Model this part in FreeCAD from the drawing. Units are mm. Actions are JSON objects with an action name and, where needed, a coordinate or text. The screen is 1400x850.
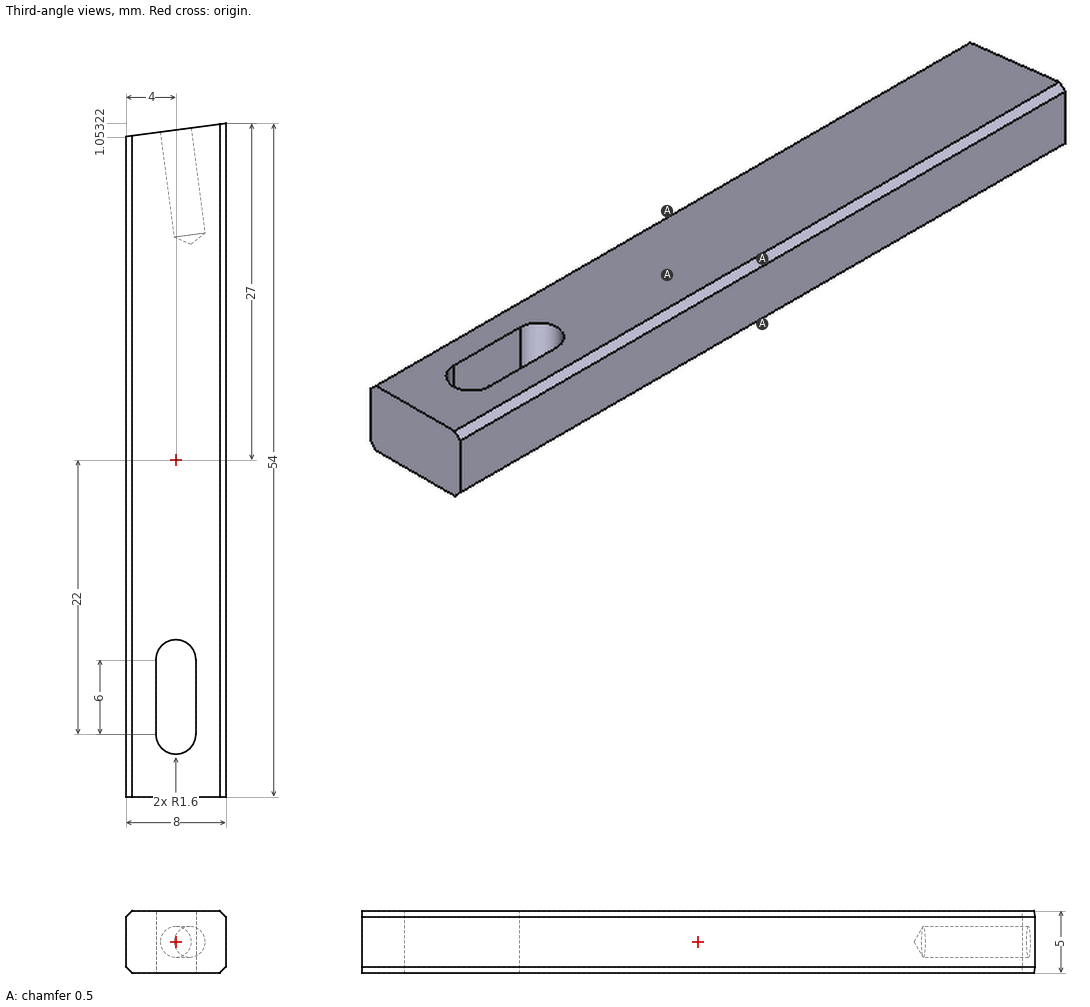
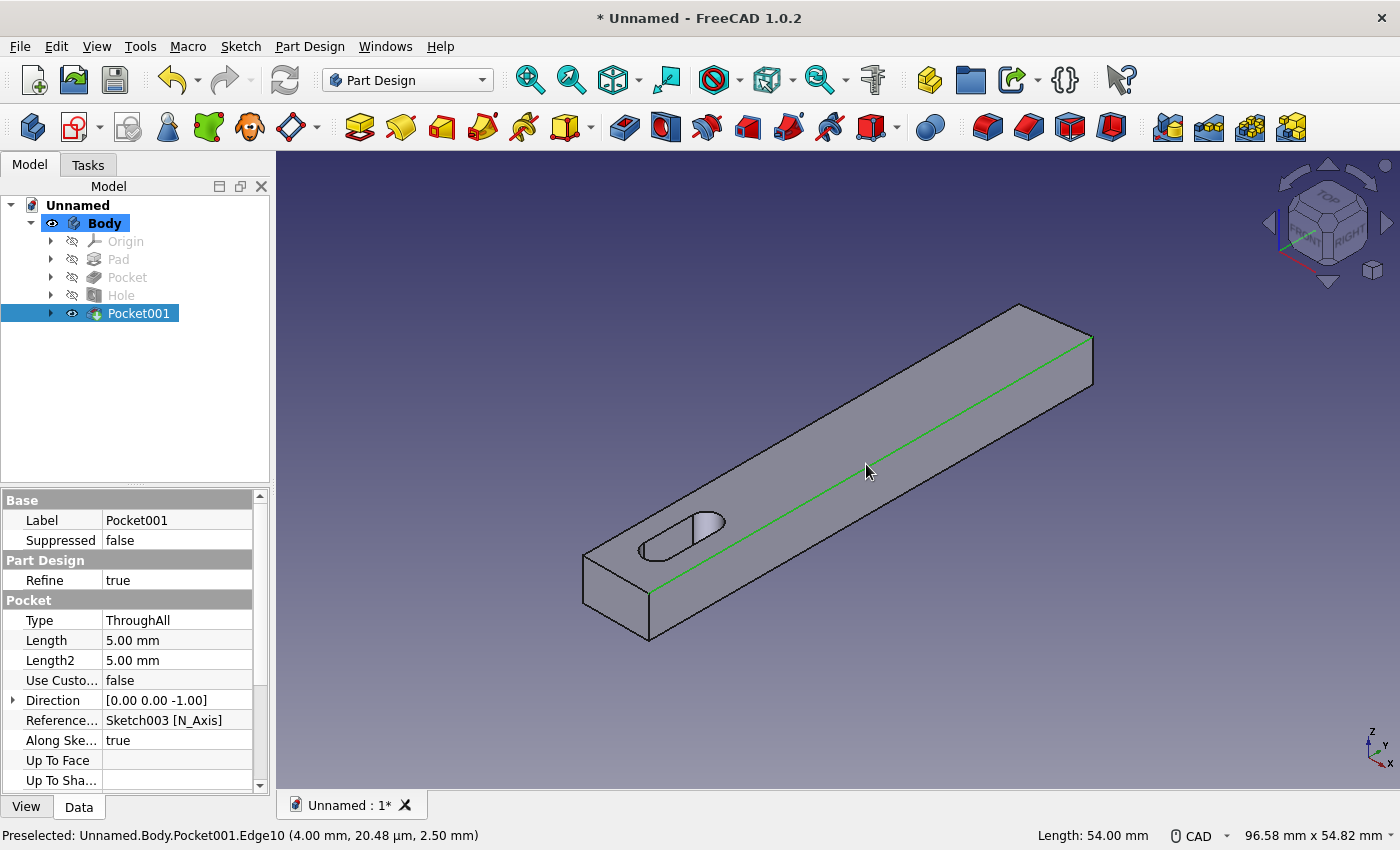
{"action": "key", "text": "2"}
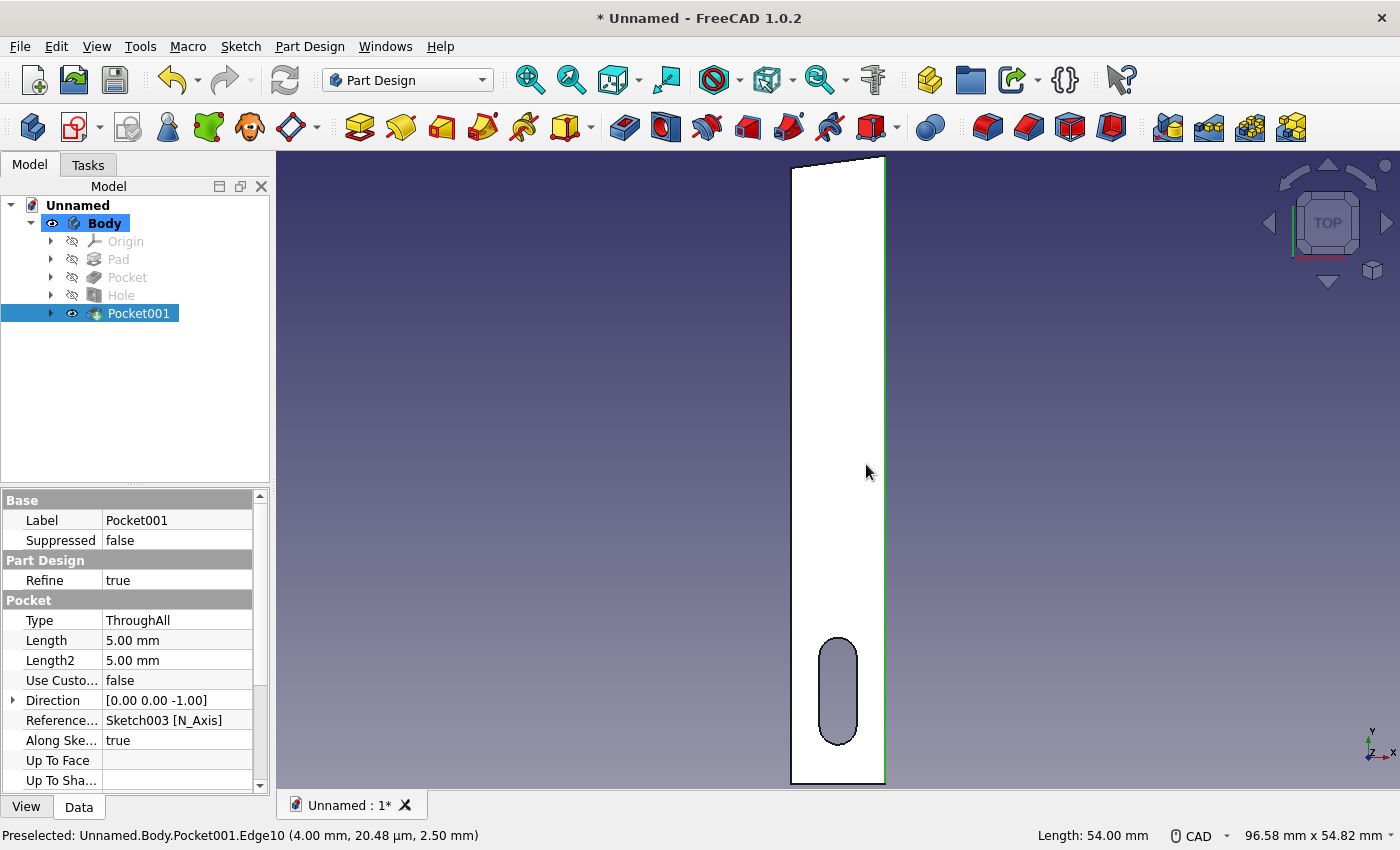
{"action": "left_click", "coordinate": [791, 475], "text": "ctrl"}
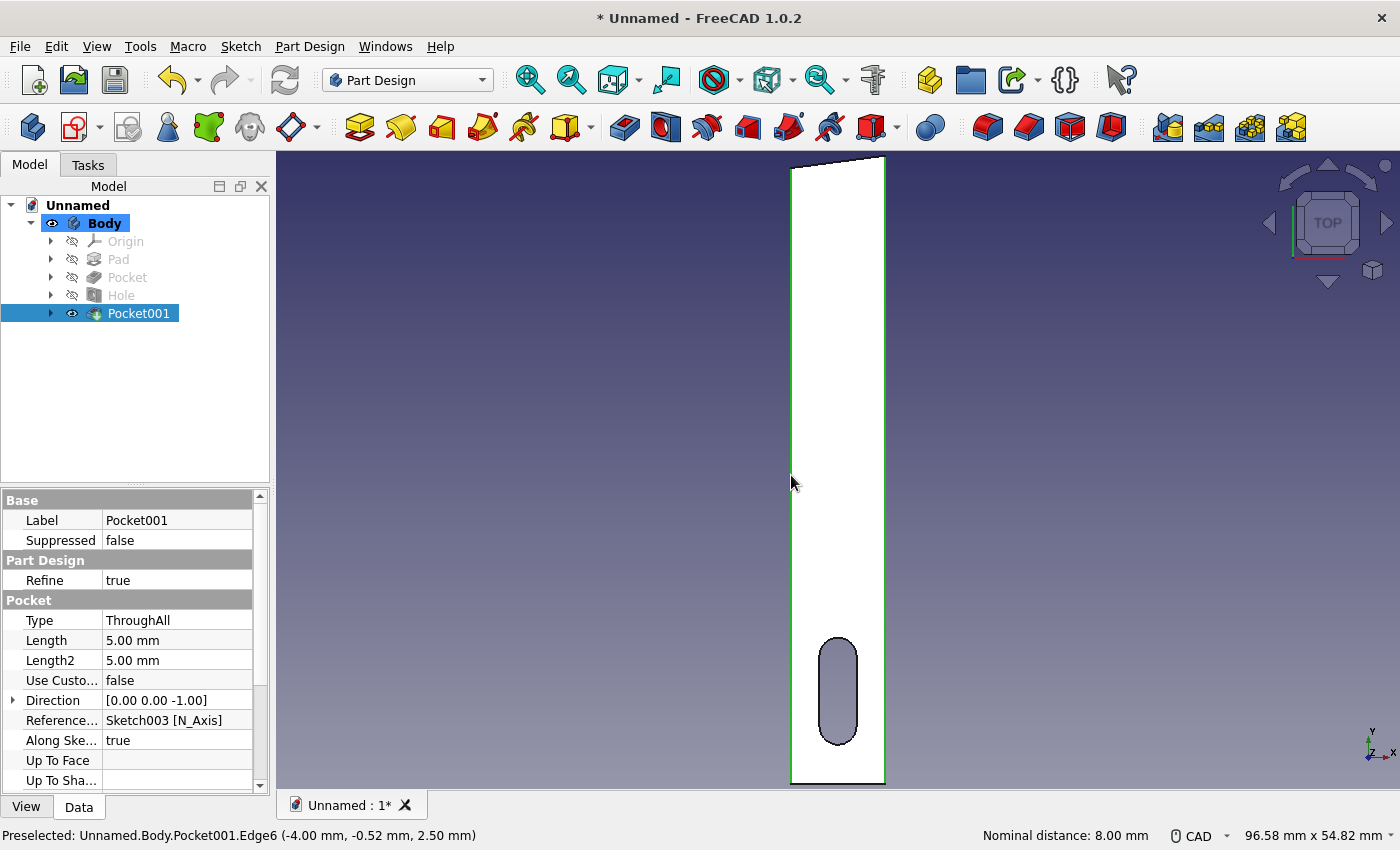
{"action": "key", "text": "0"}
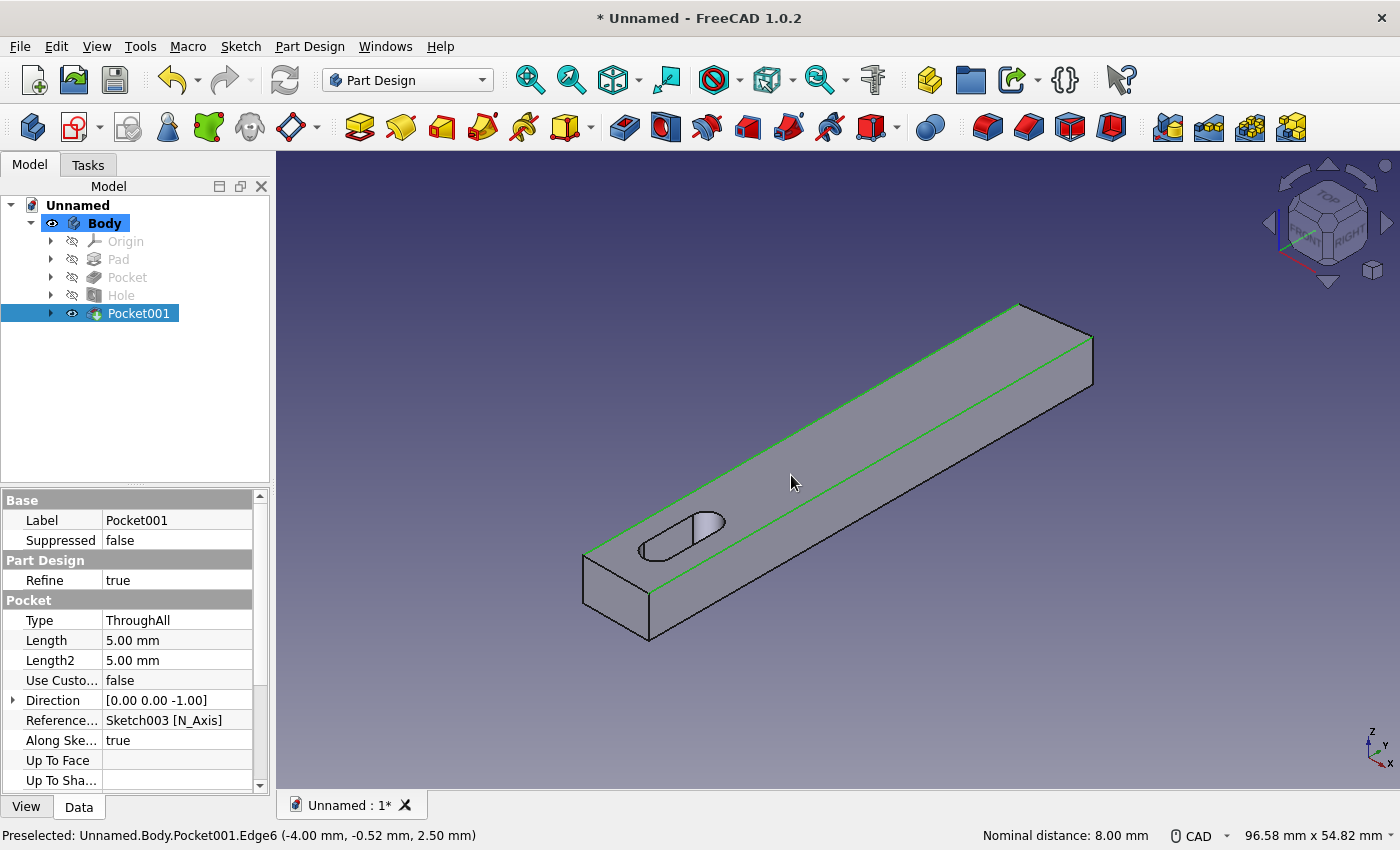
{"action": "key", "text": "1"}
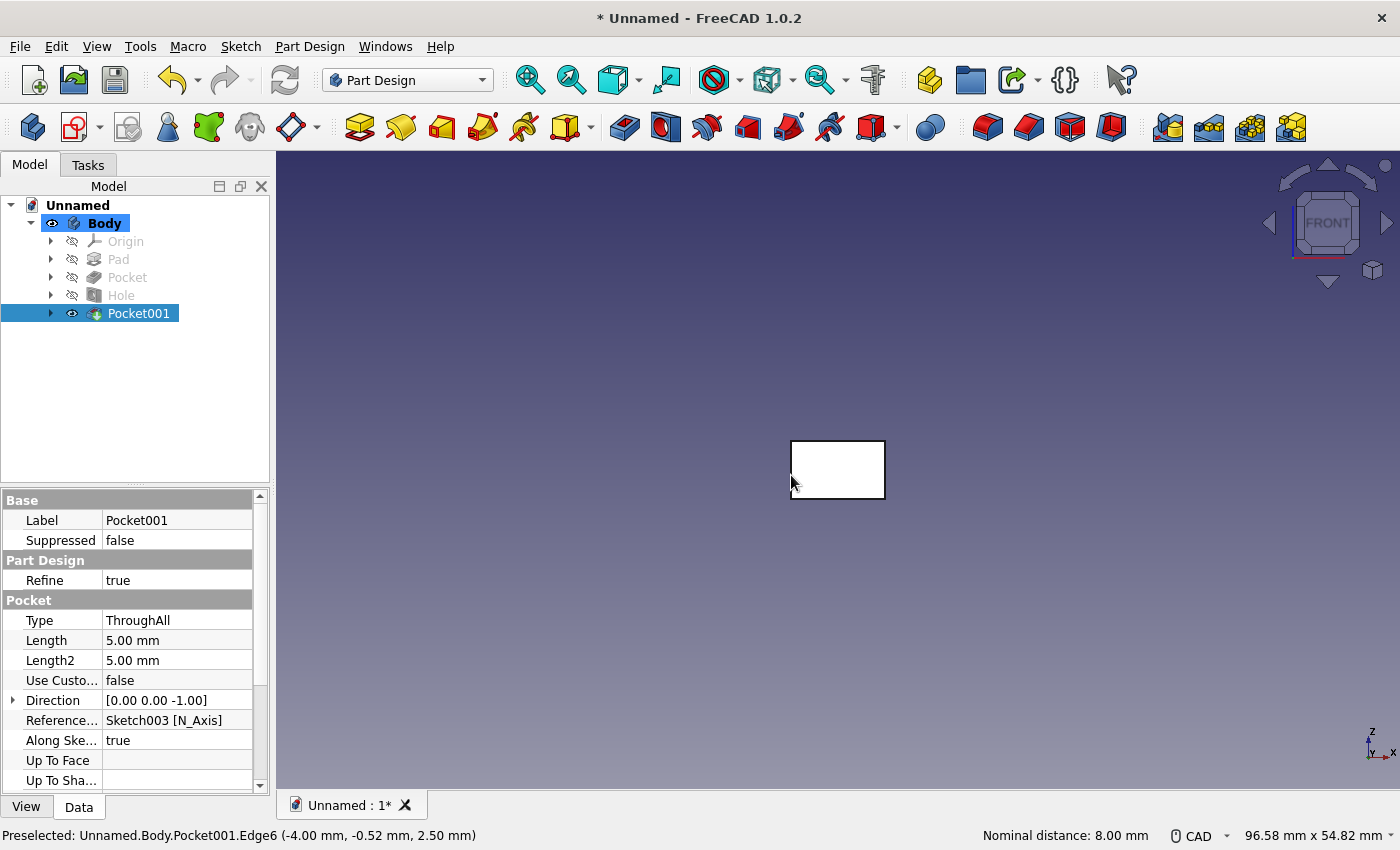
{"action": "left_click", "coordinate": [531, 80]}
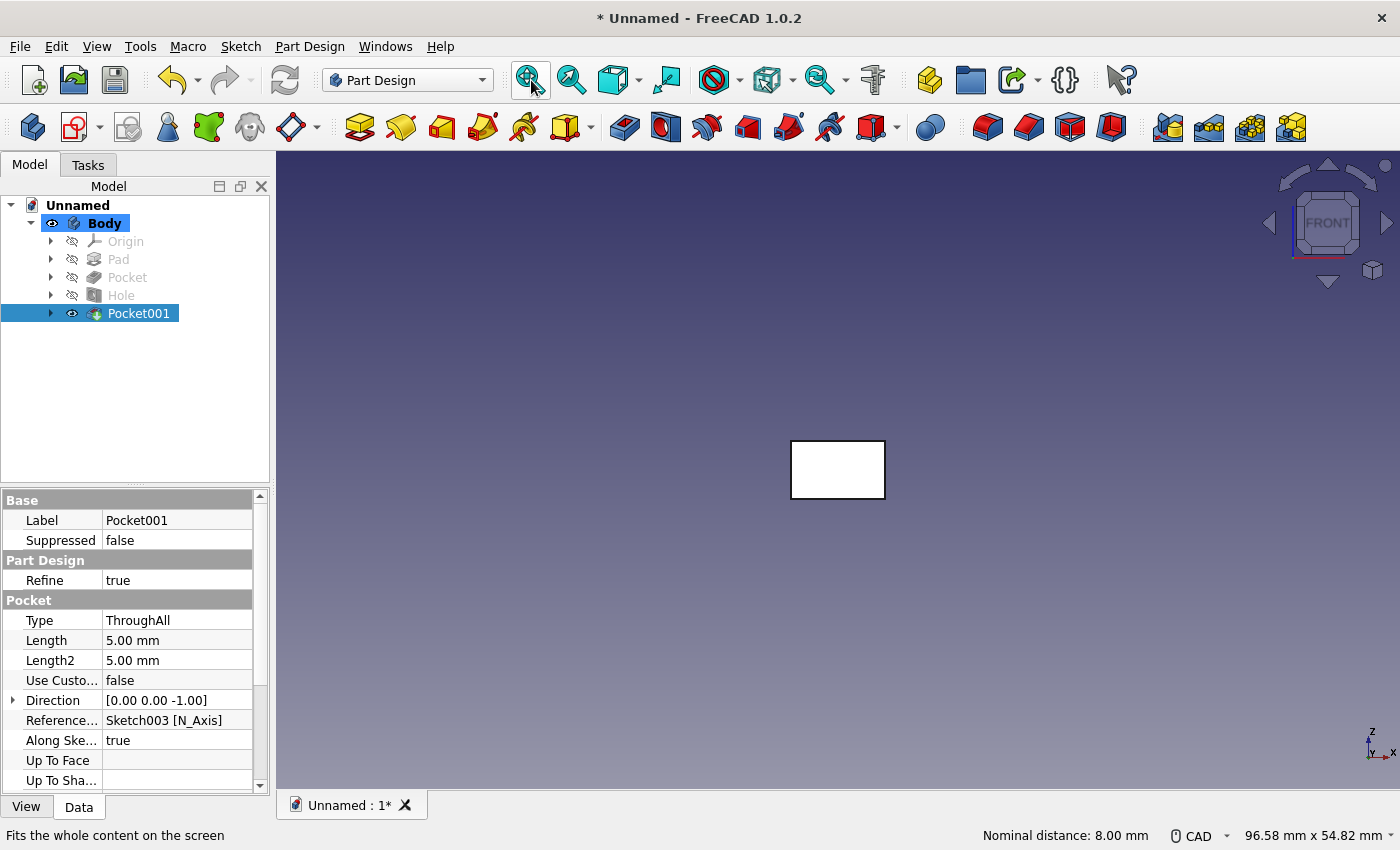
{"action": "key", "text": "3"}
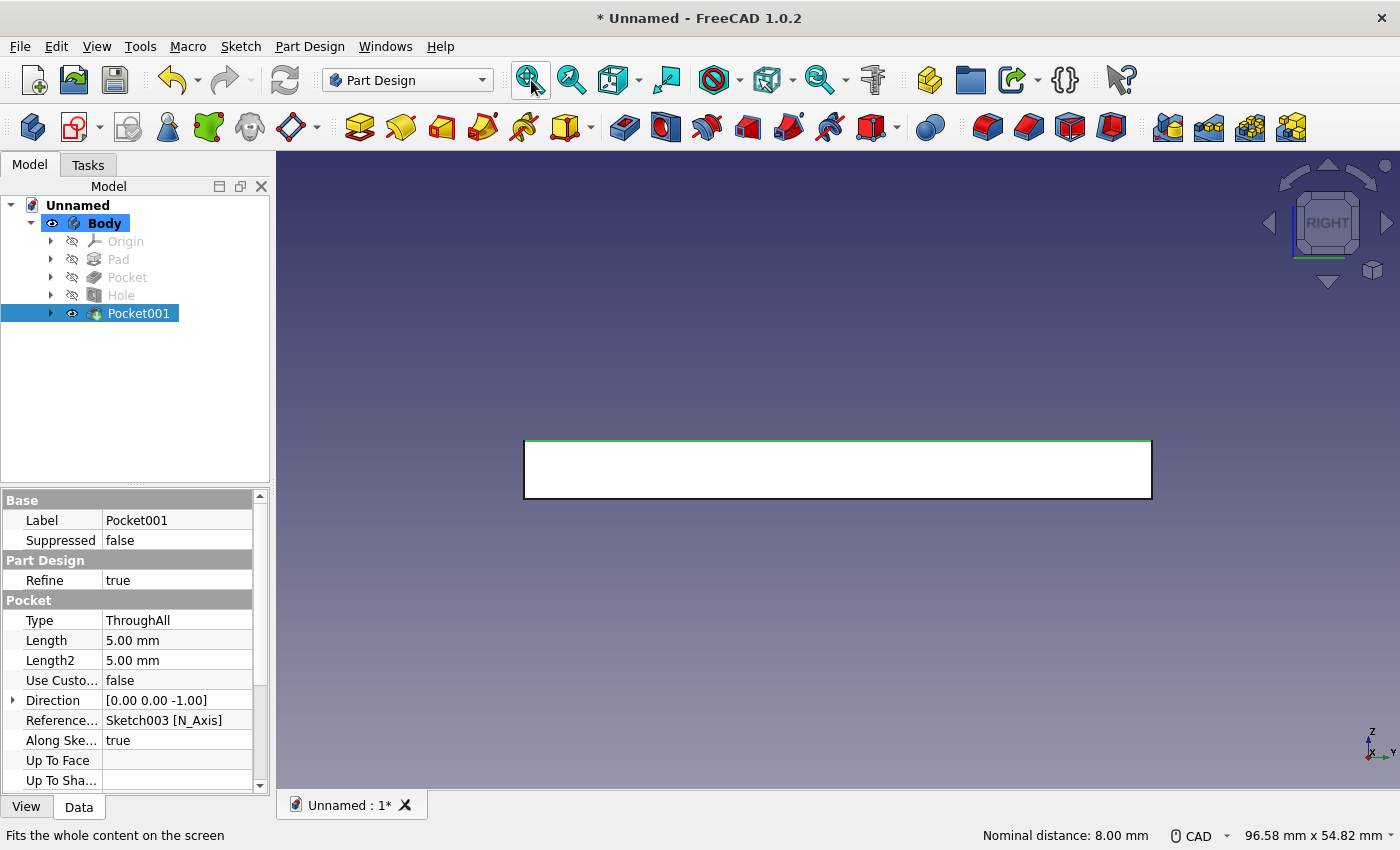
{"action": "left_click", "coordinate": [838, 498], "text": "ctrl"}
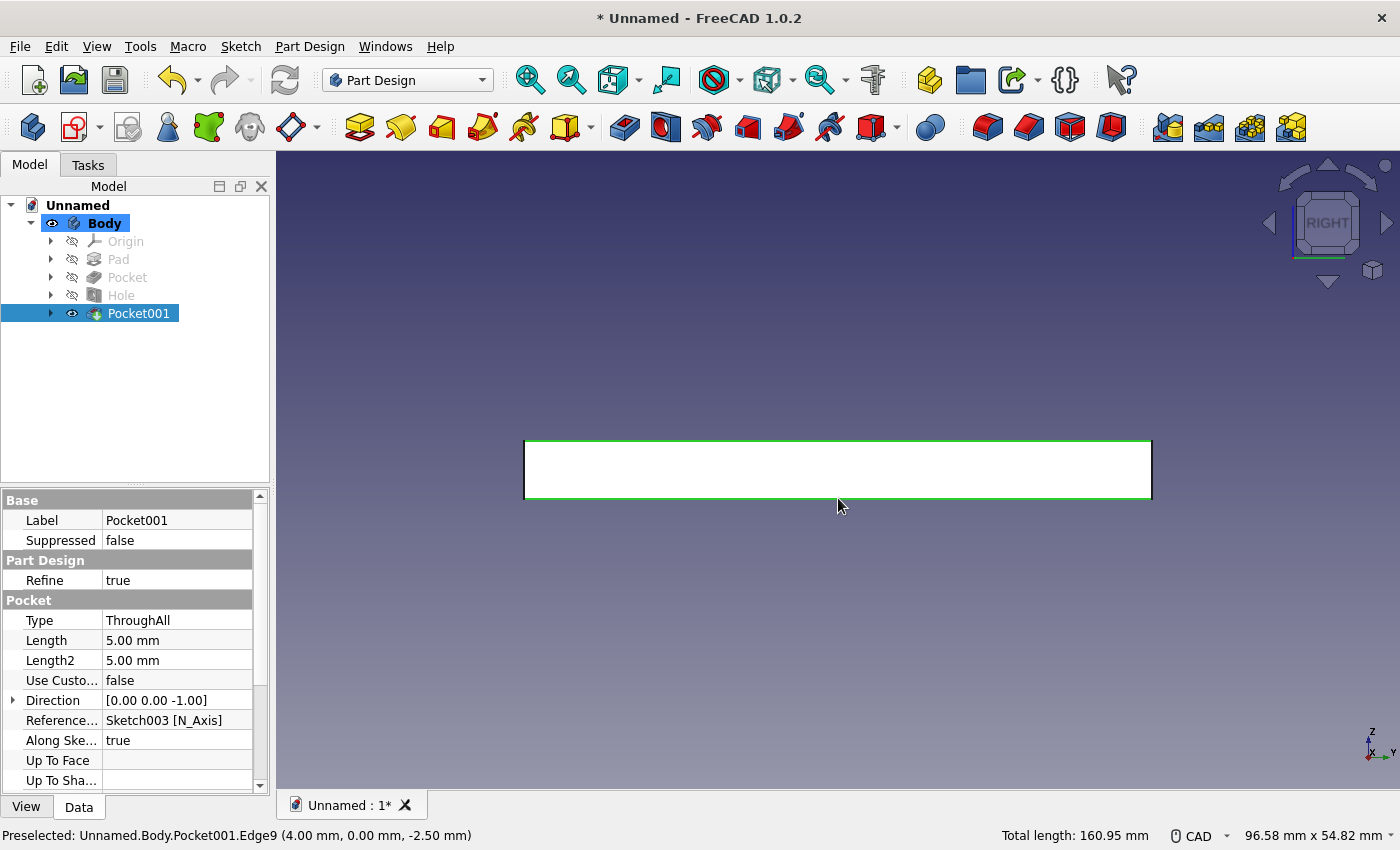
{"action": "key", "text": "5"}